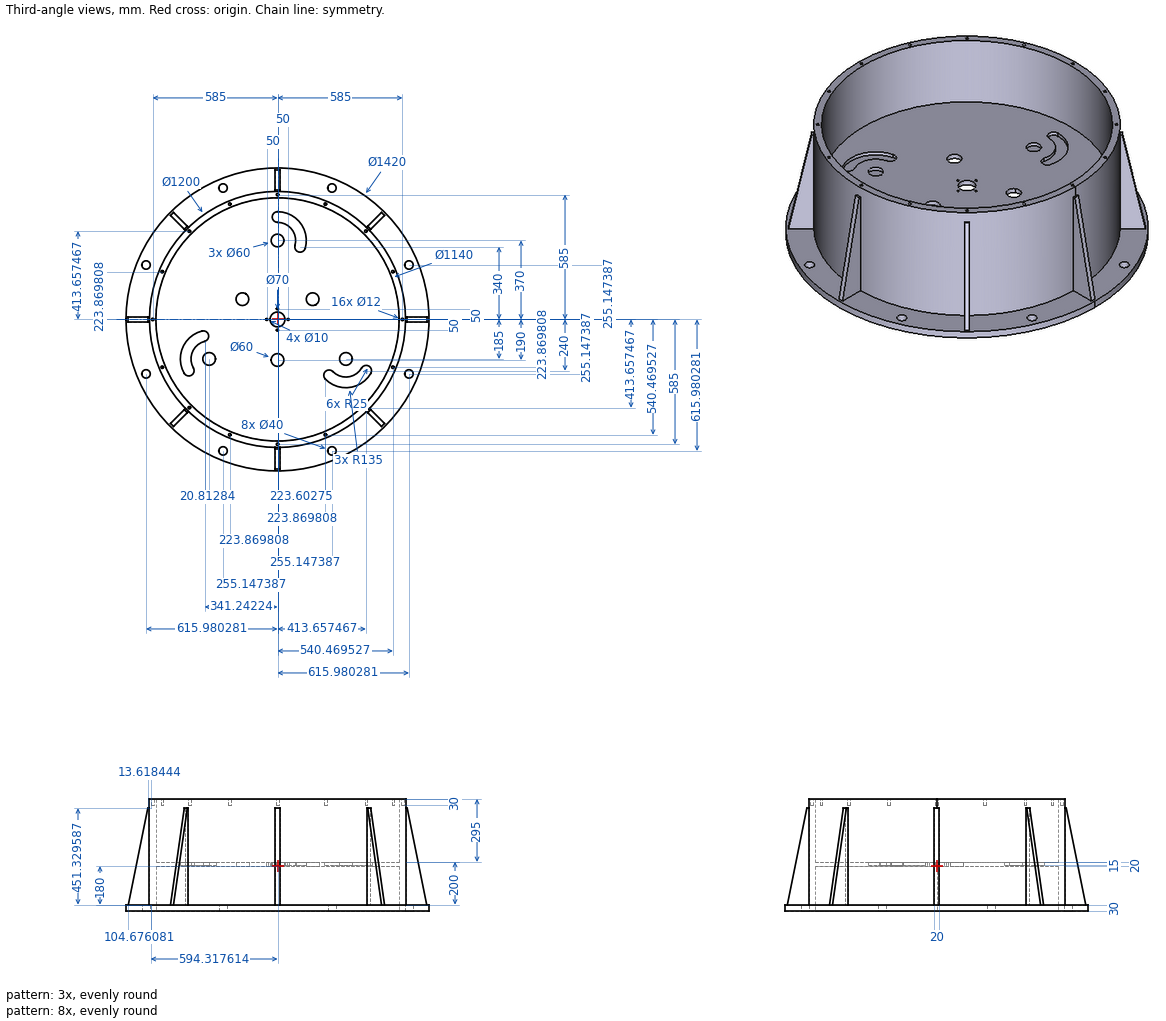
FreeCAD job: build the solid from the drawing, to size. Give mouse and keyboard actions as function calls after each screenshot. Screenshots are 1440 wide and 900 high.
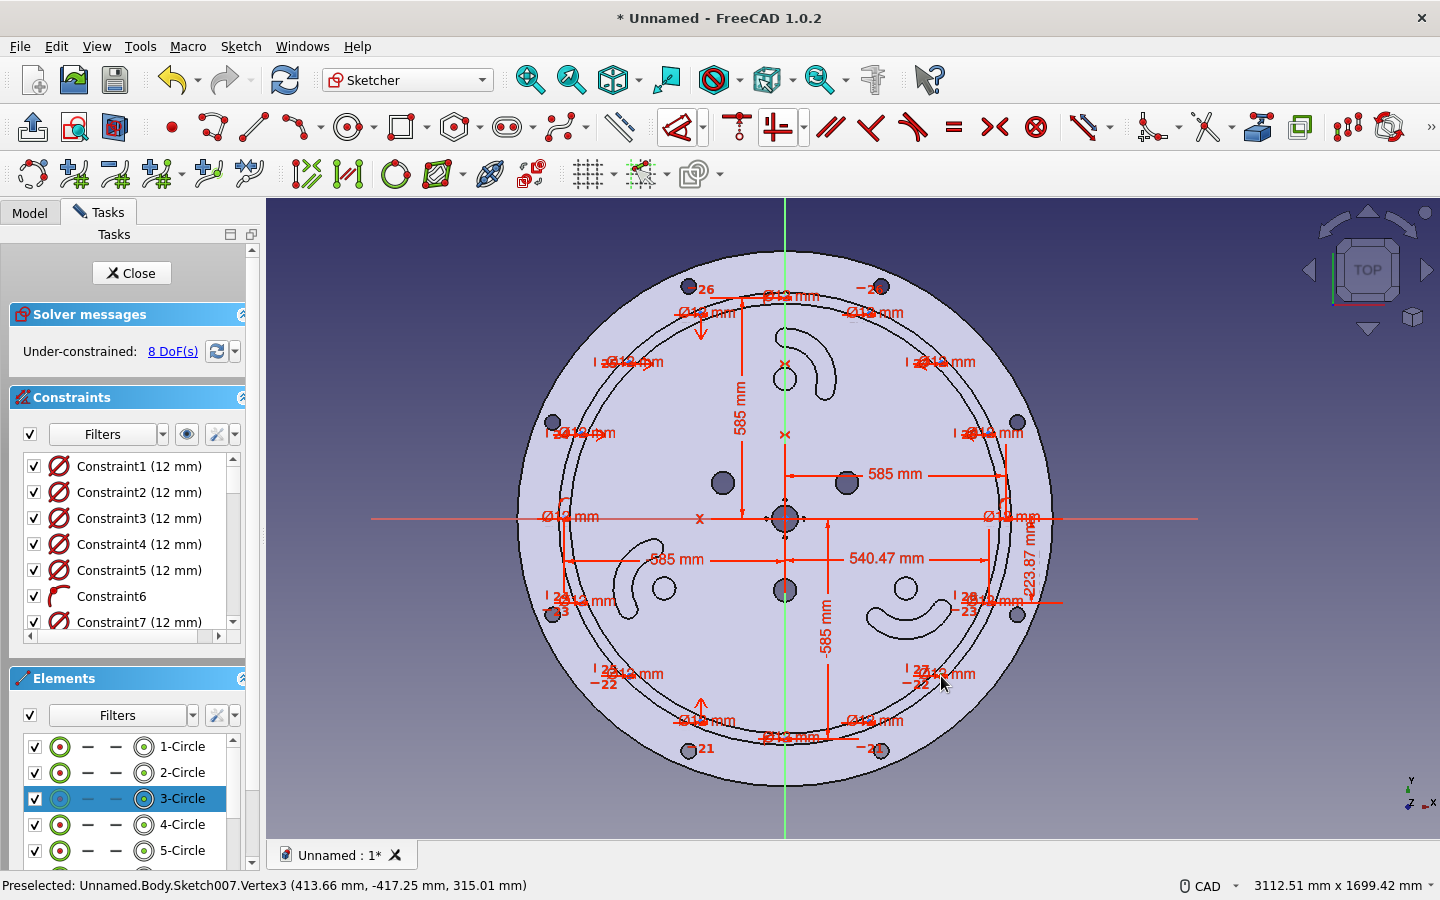
key(l)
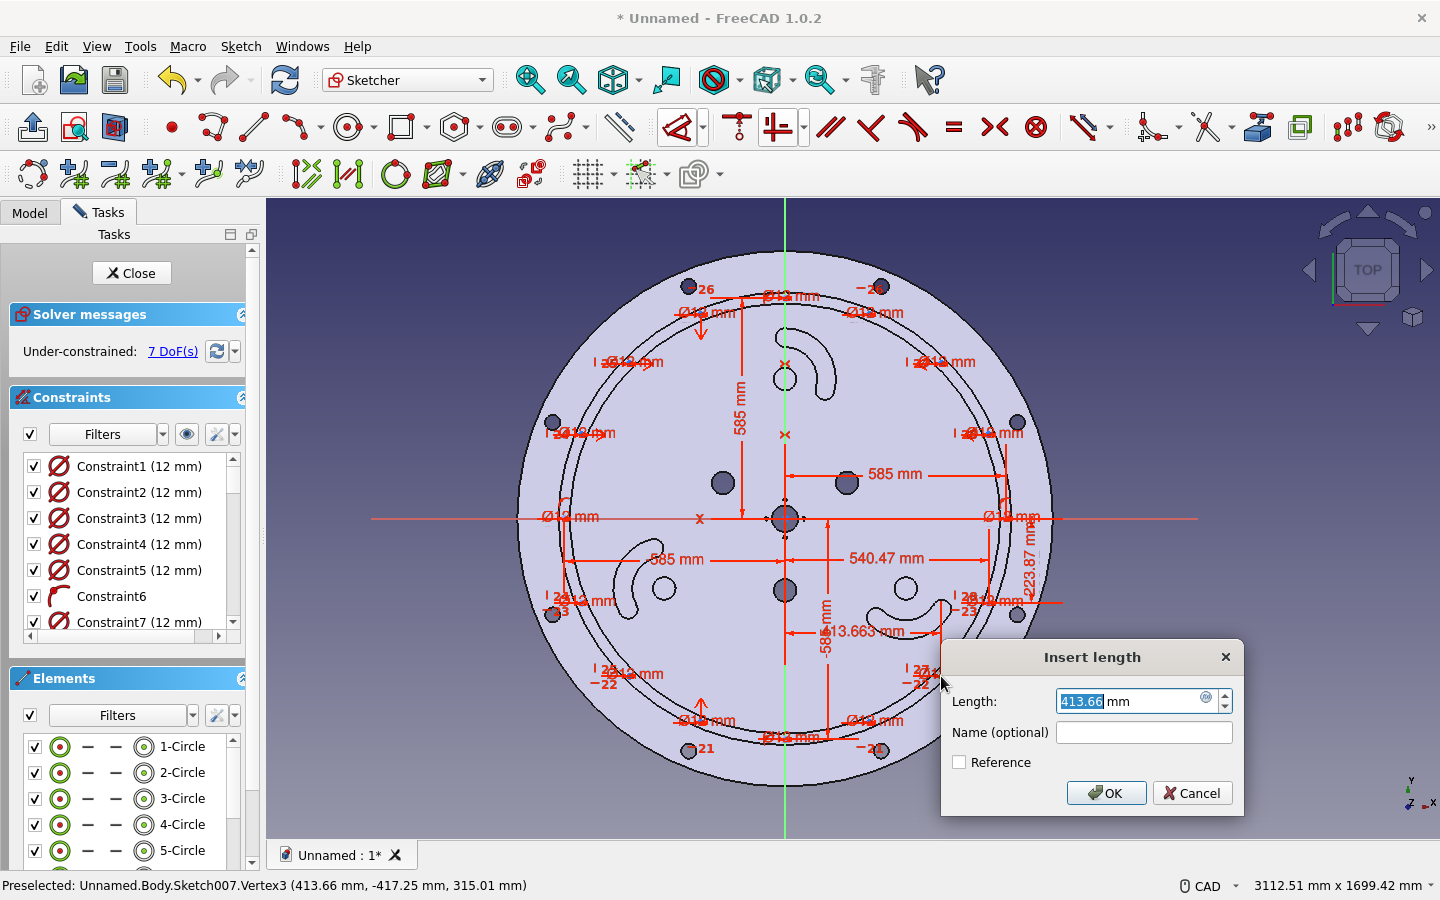
text(413.657467)
key(Return)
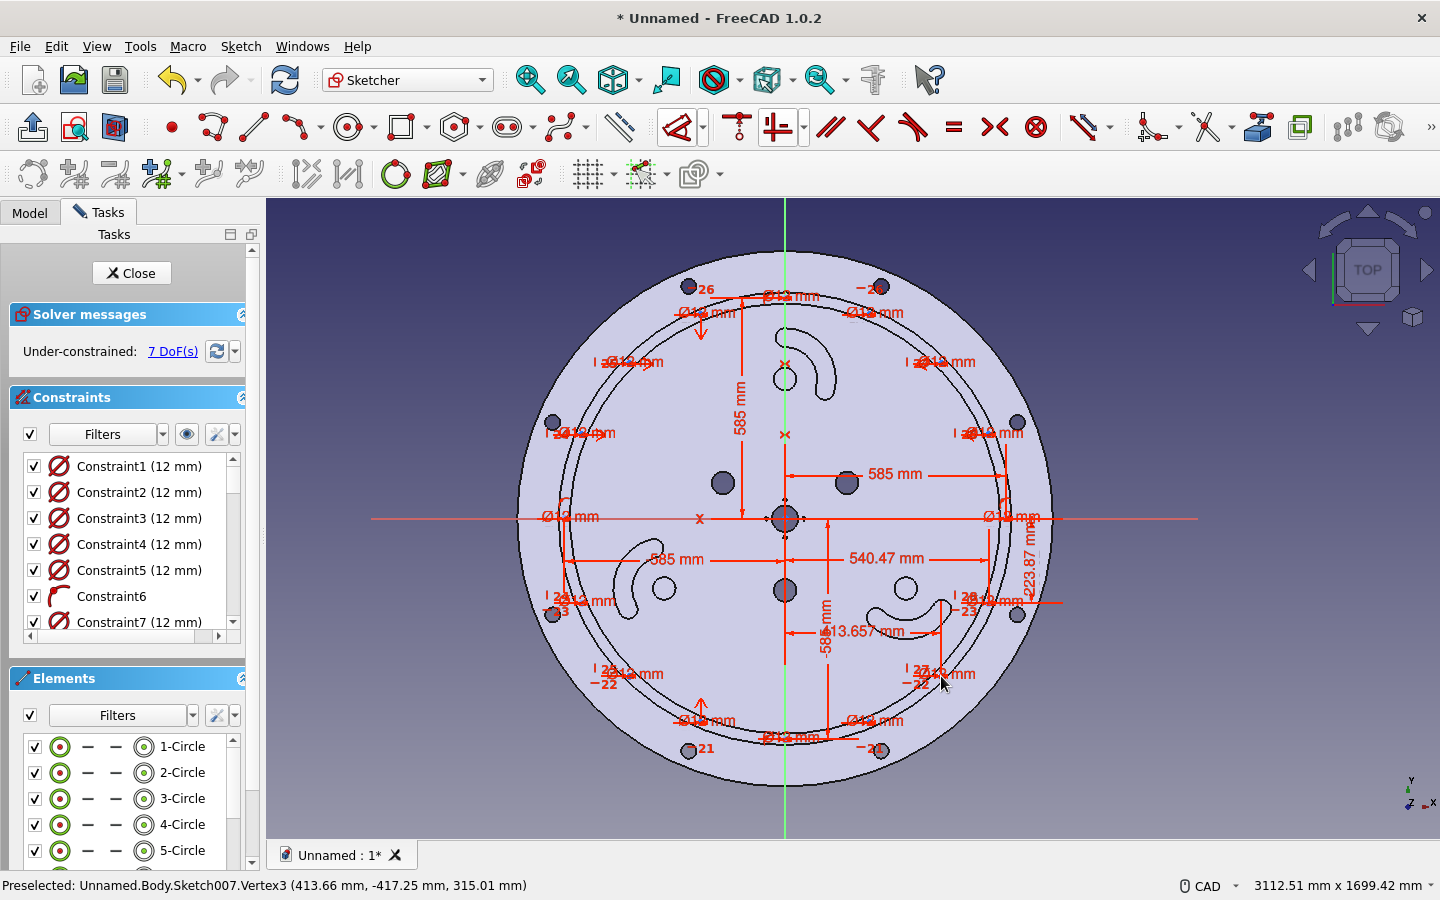
click(941, 676)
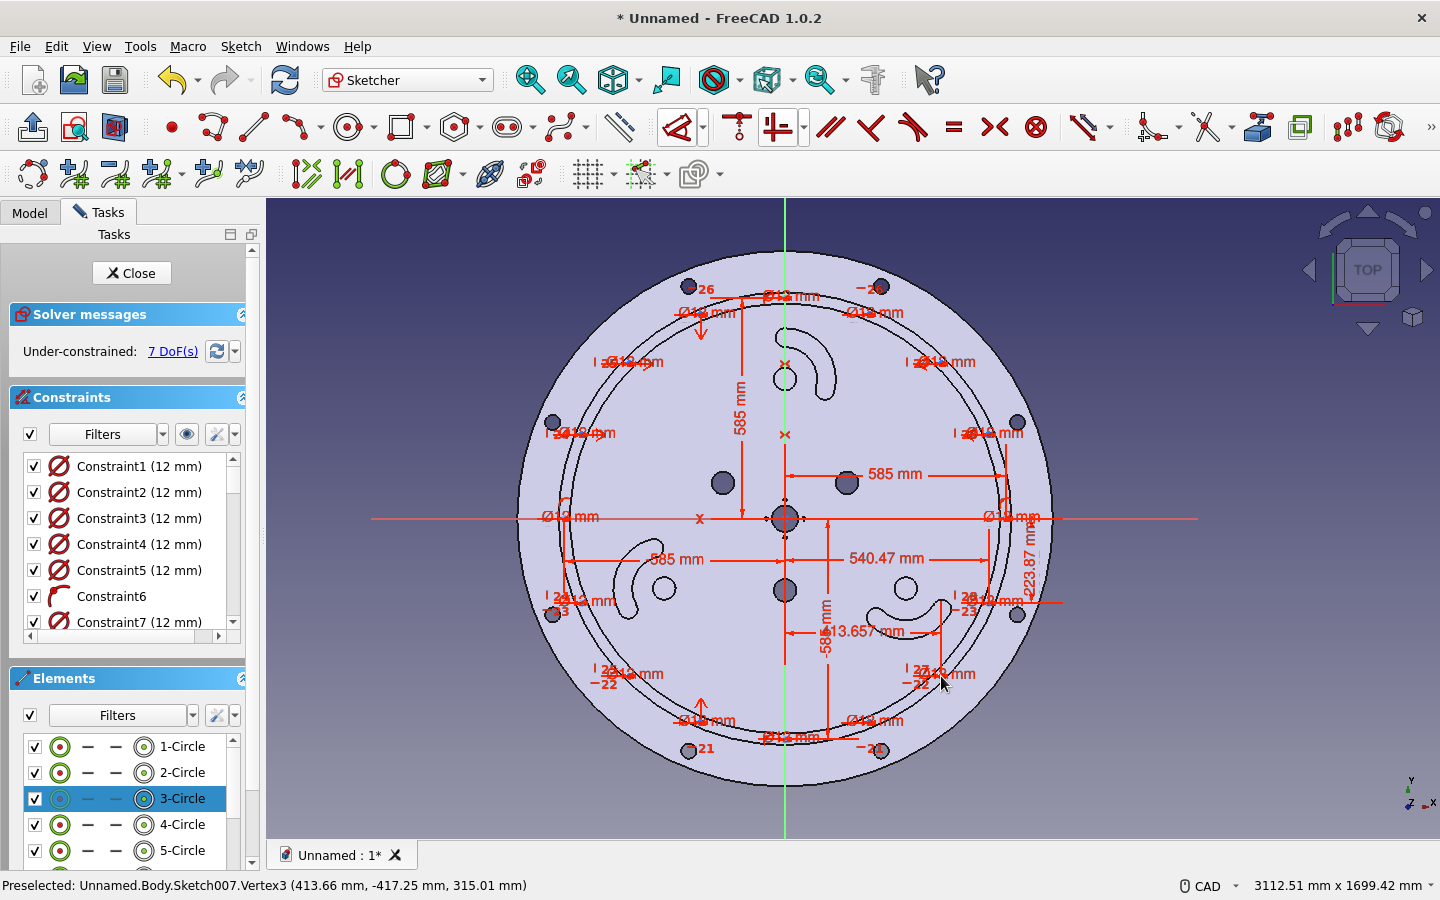
key(i)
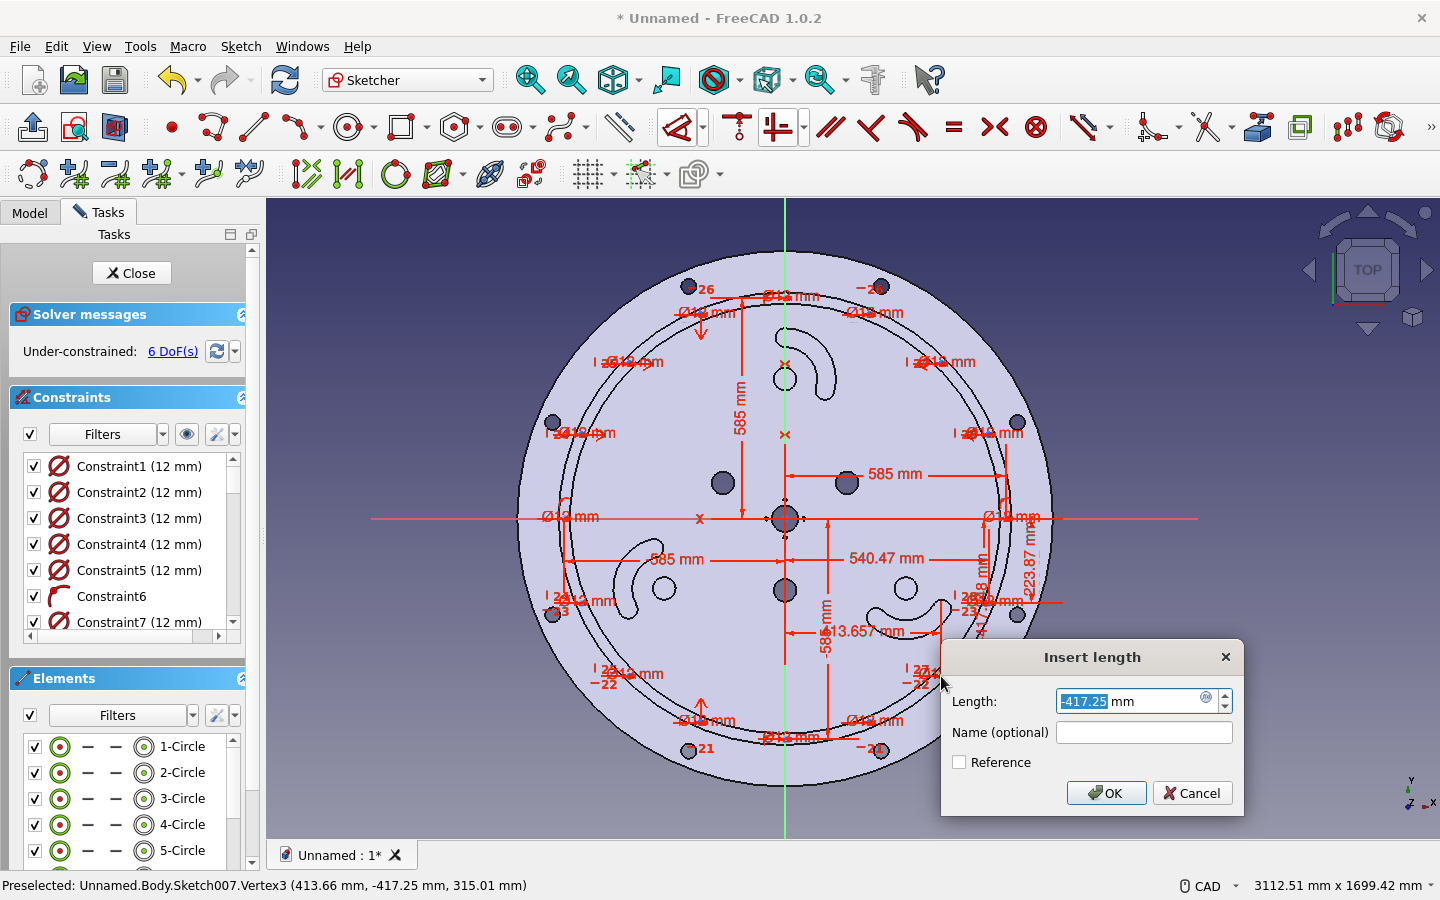
text(-413.657467)
key(Return)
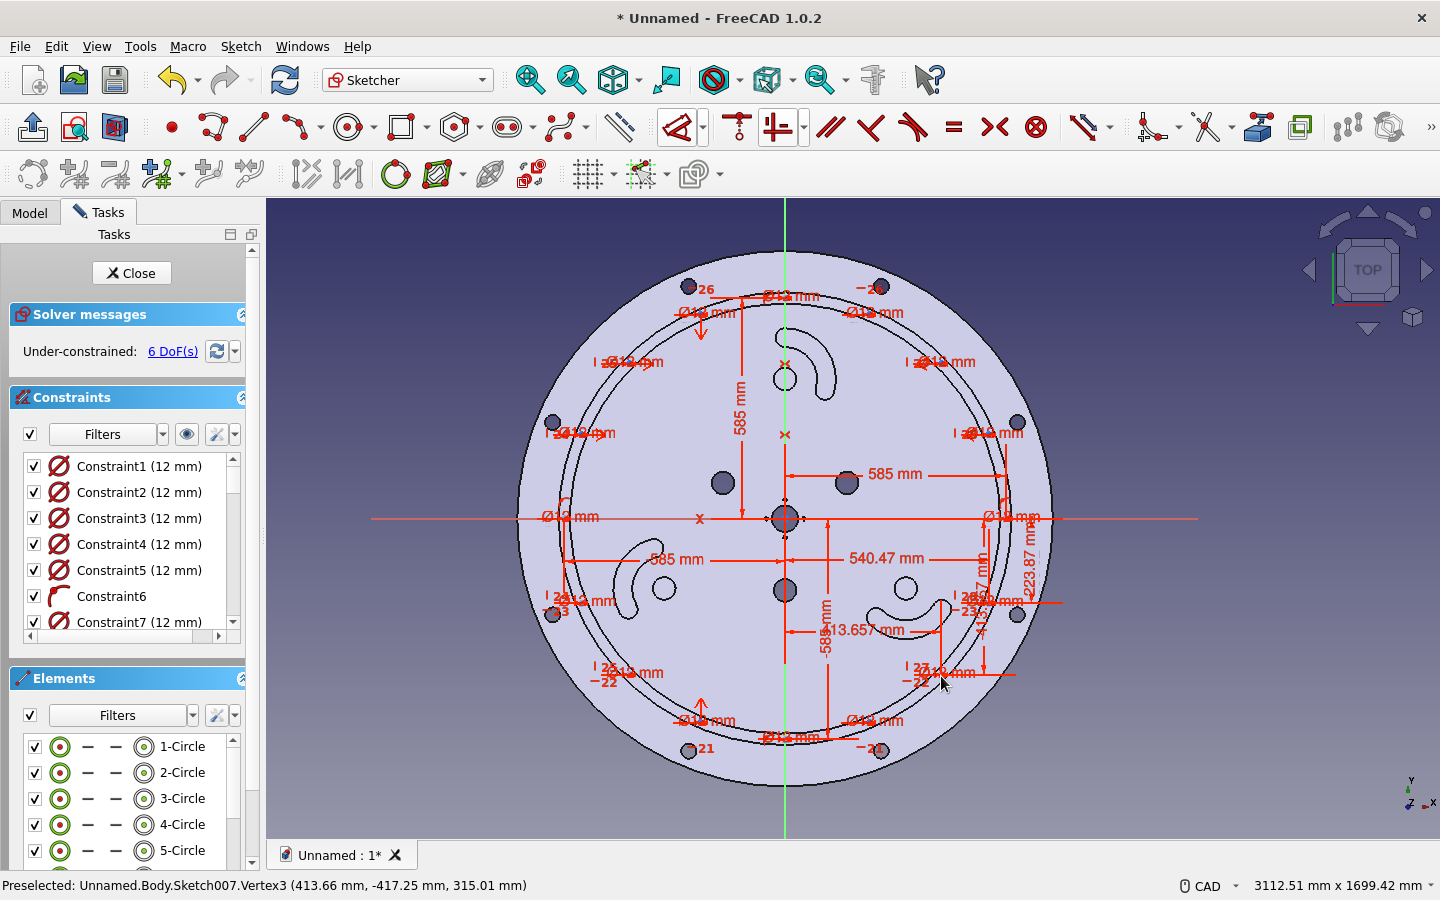
click(869, 723)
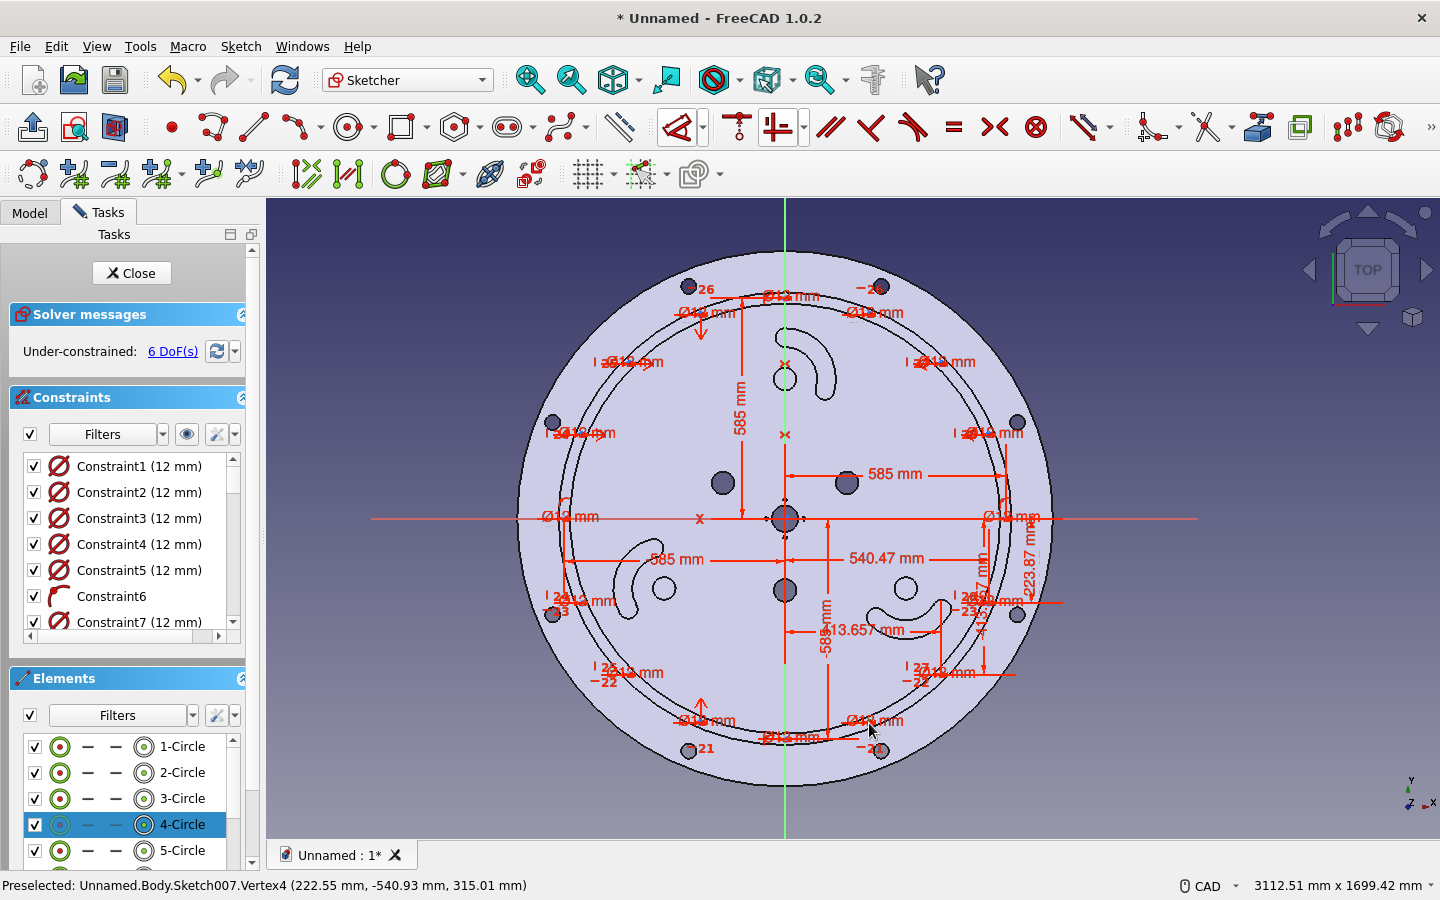
click(702, 128)